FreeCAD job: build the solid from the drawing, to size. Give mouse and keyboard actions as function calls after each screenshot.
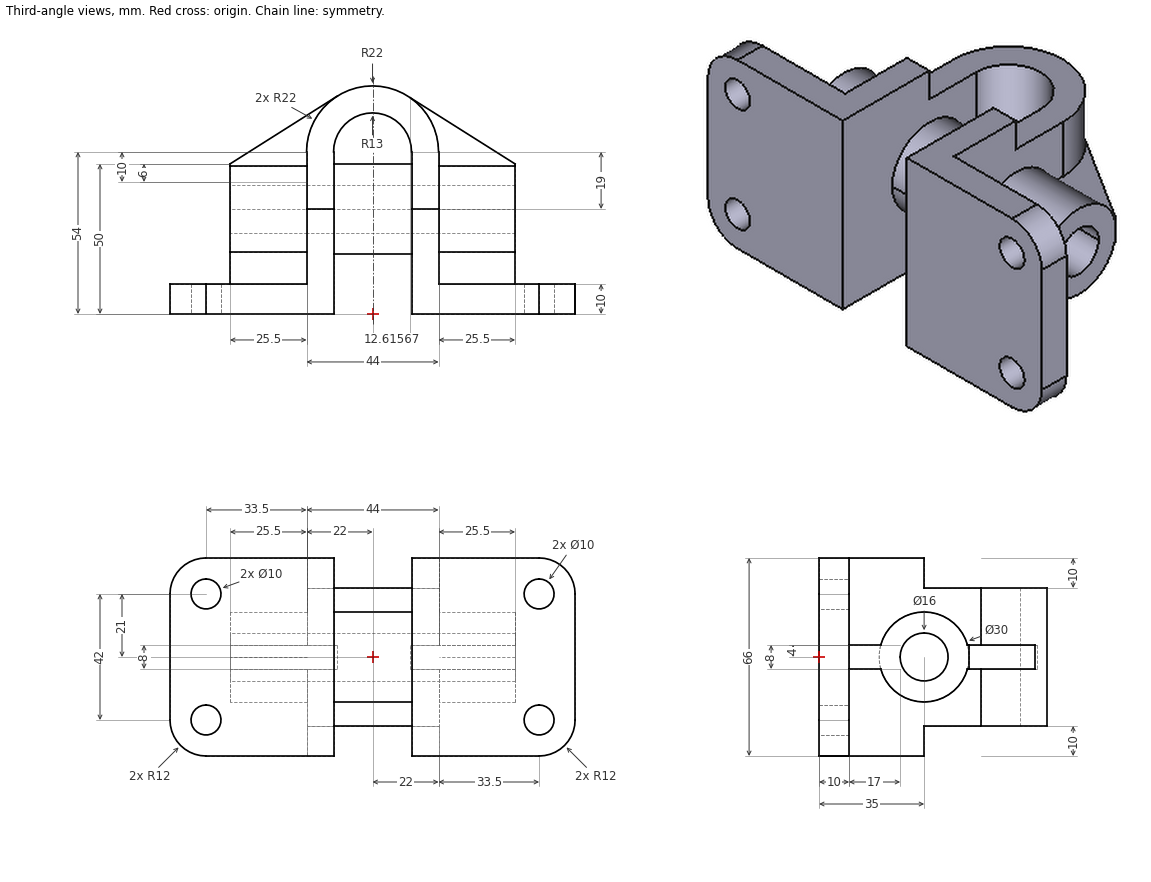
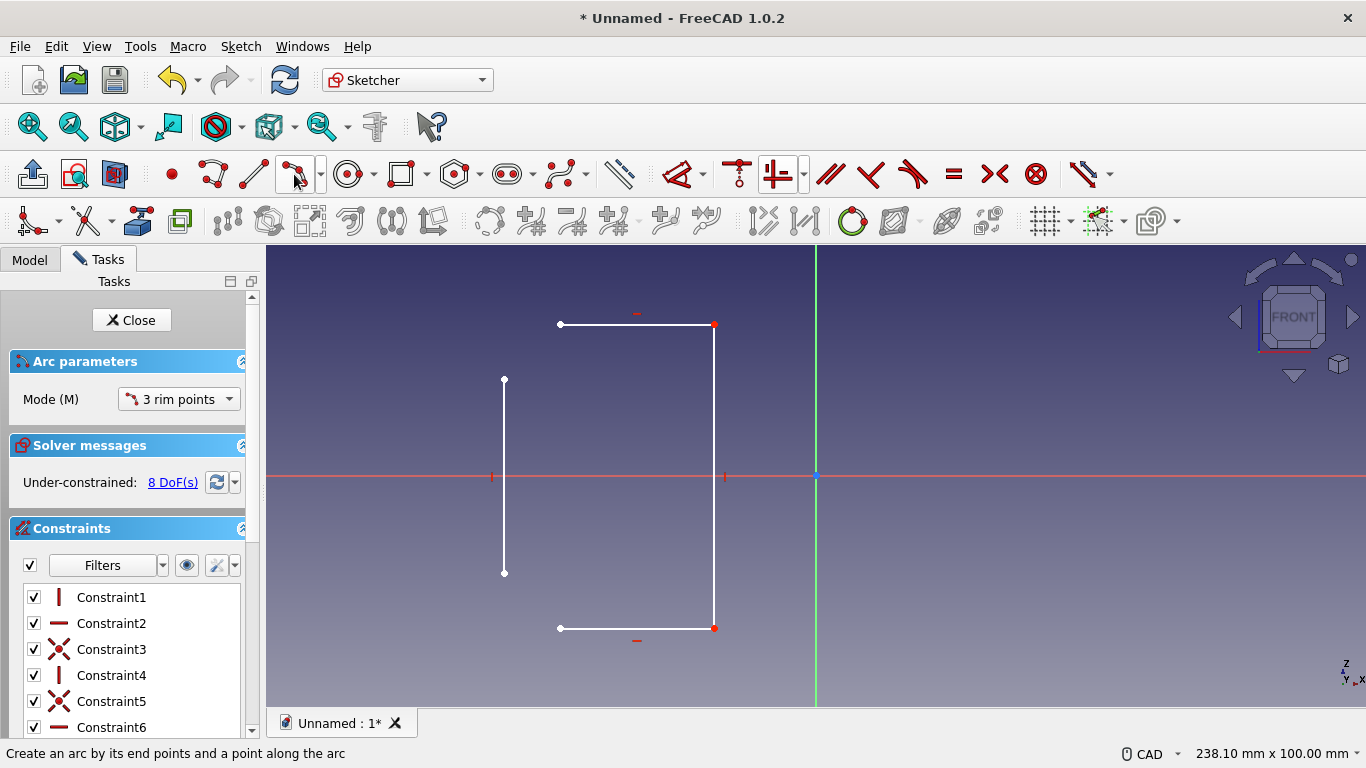
click(504, 380)
click(560, 325)
click(520, 340)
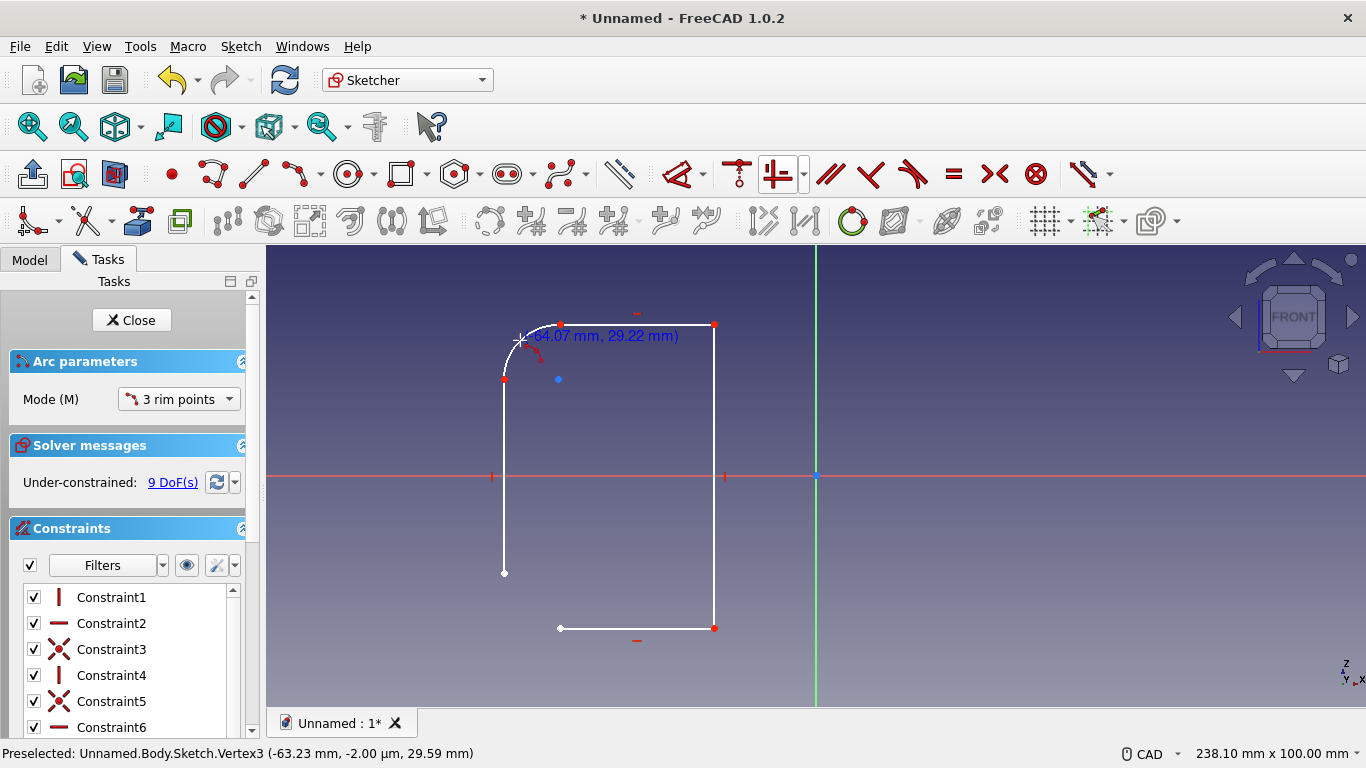
click(560, 629)
click(504, 574)
click(520, 612)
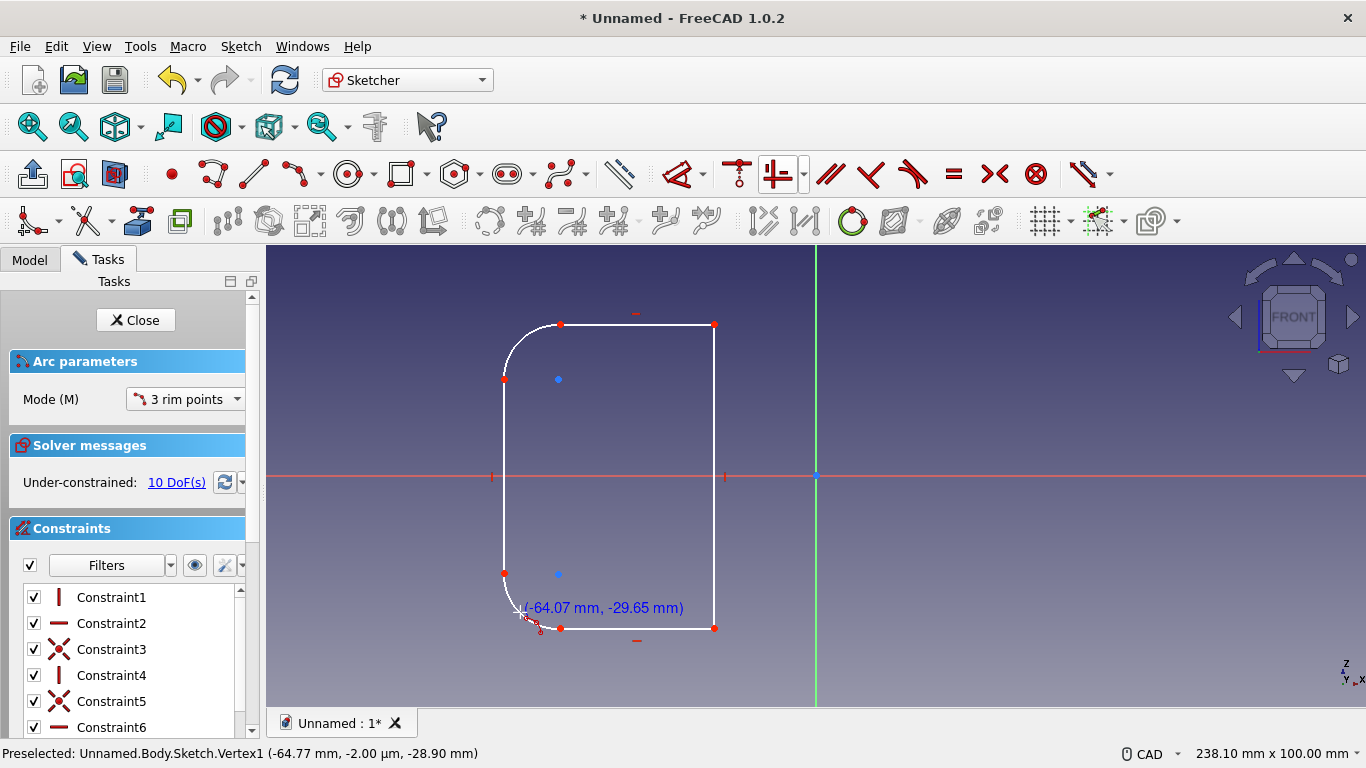
click(348, 174)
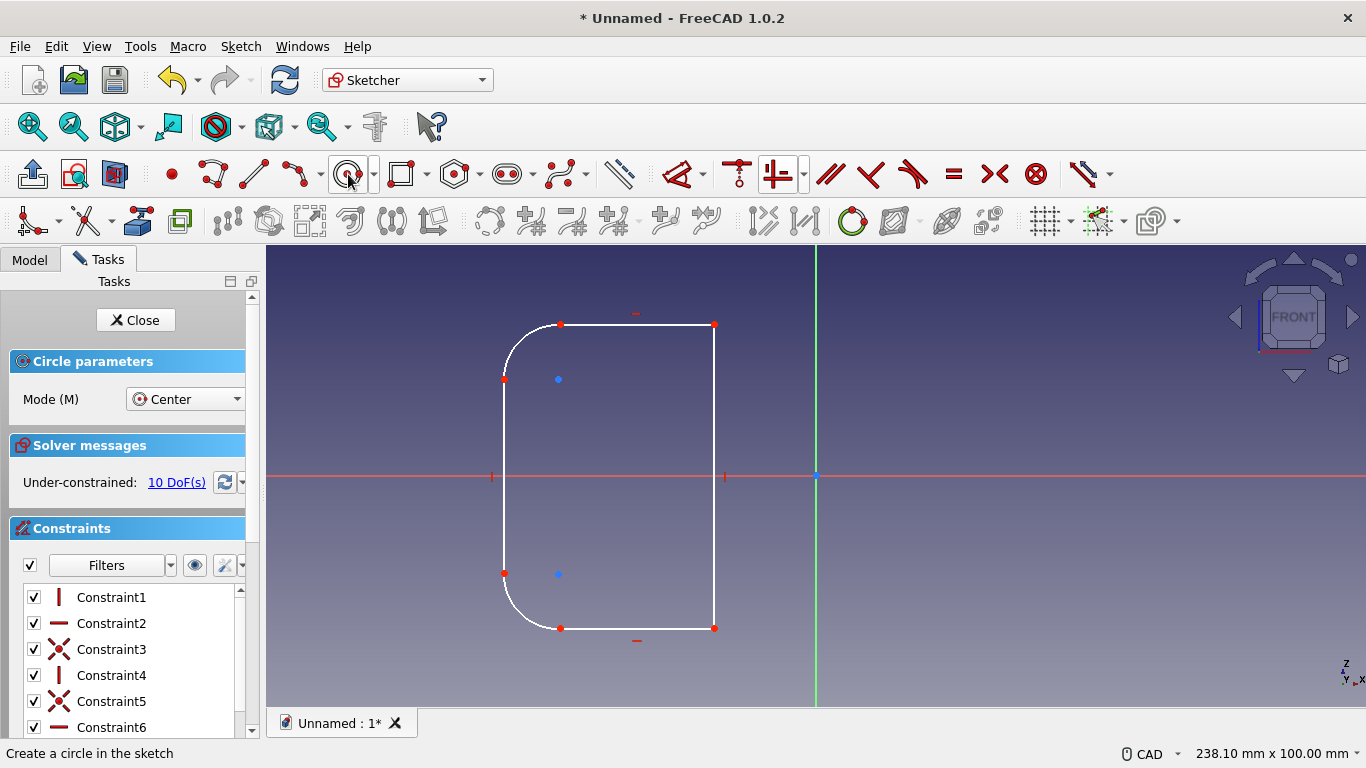
click(560, 379)
move(576, 363)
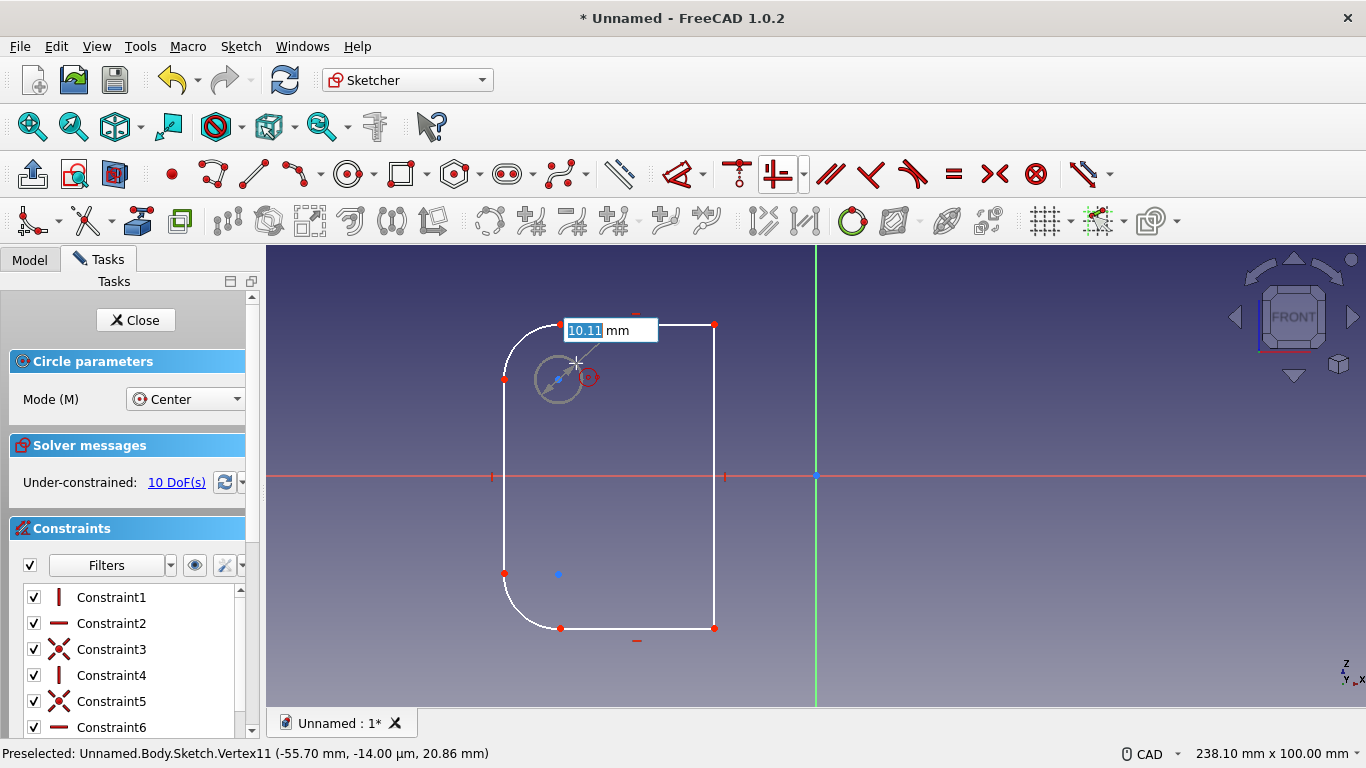
text(10)
key(Return)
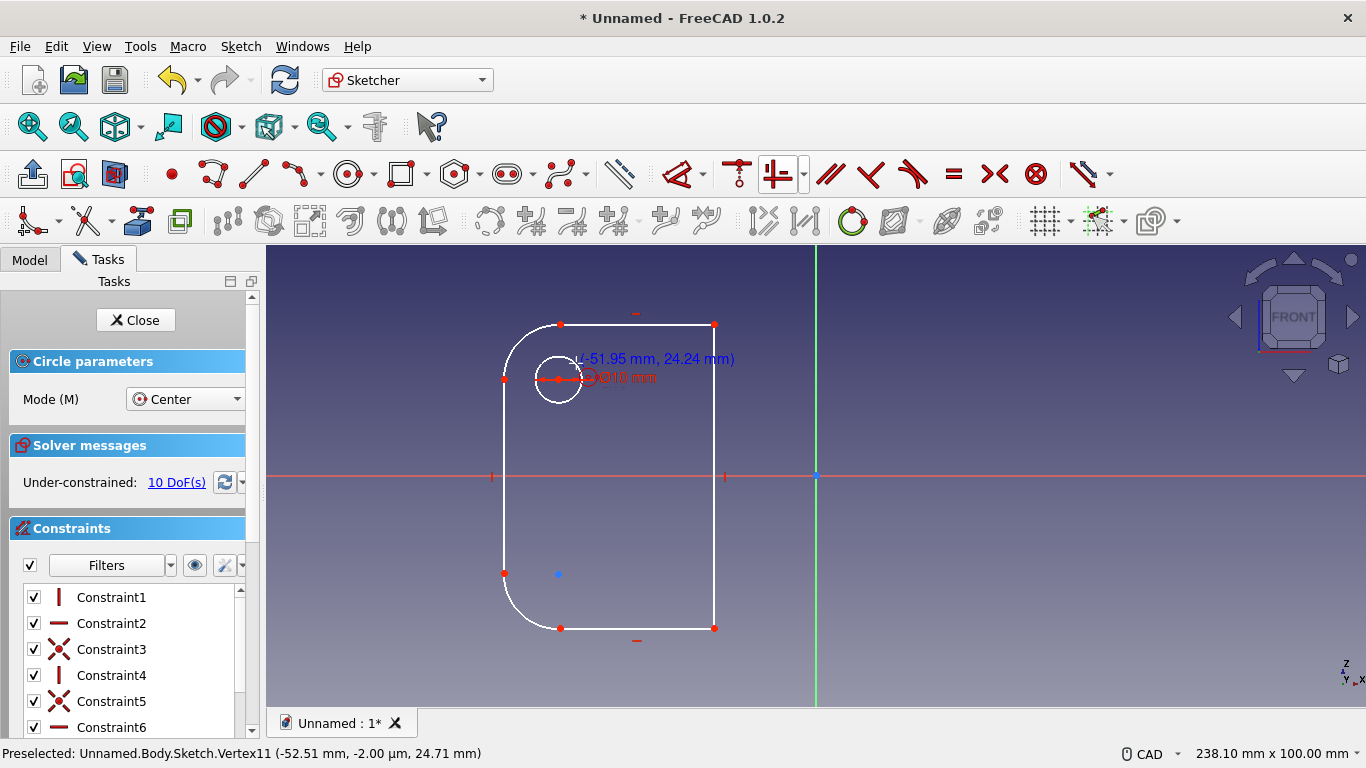
click(560, 573)
move(576, 557)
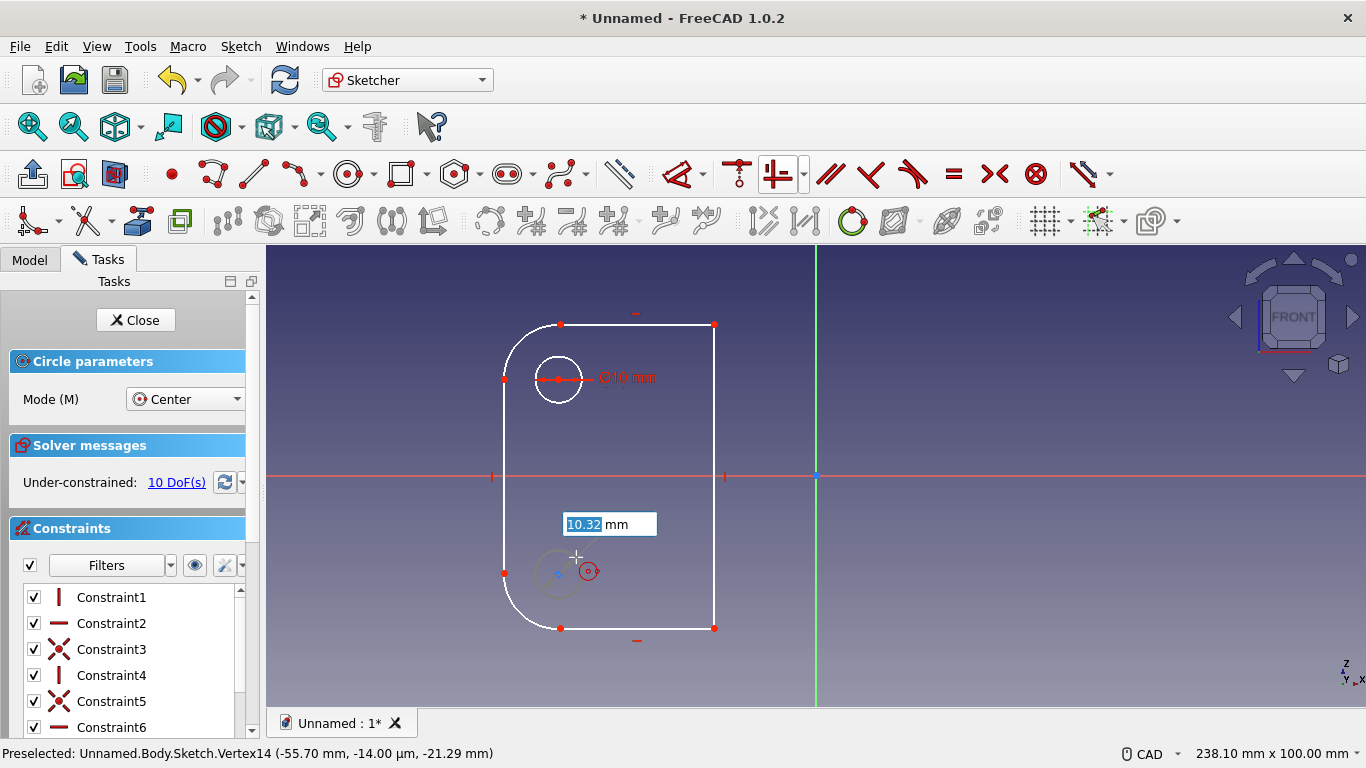
text(10)
key(Return)
key(Escape)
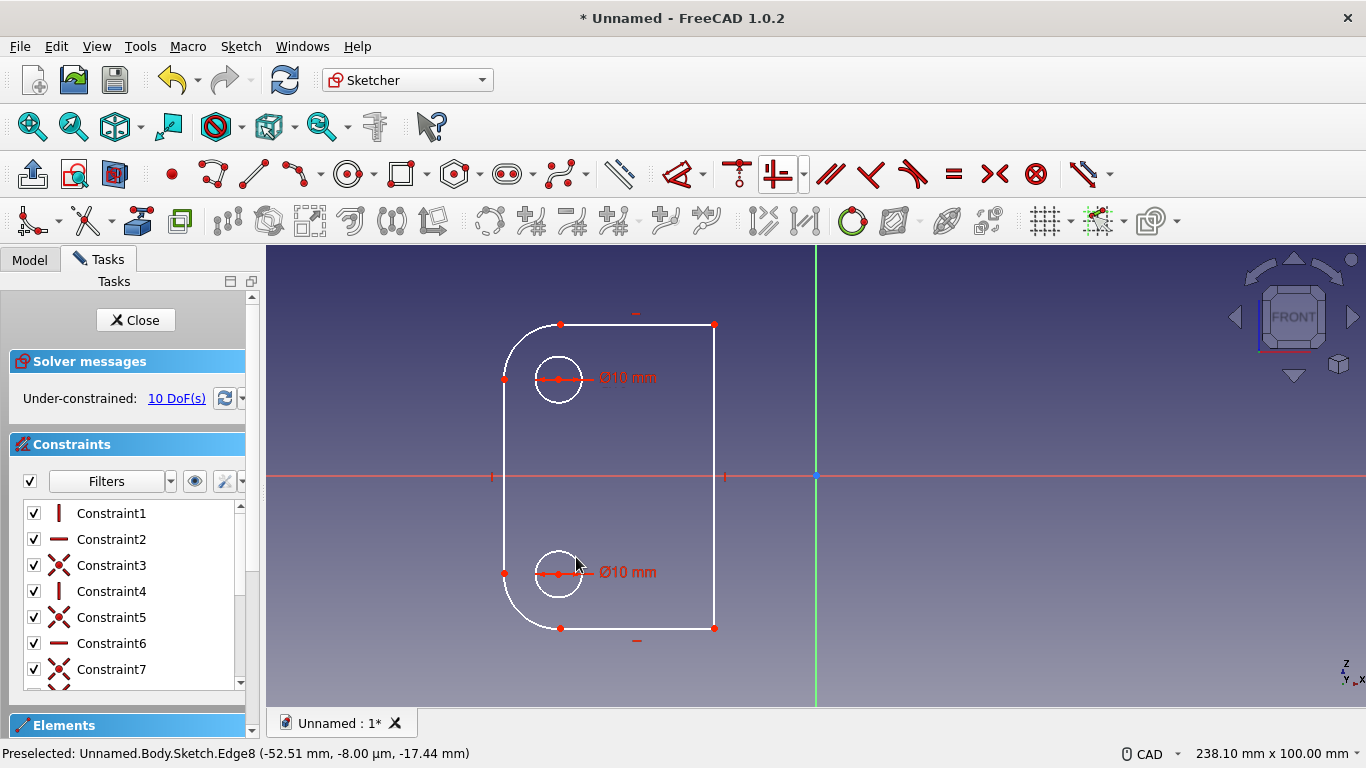
click(504, 516)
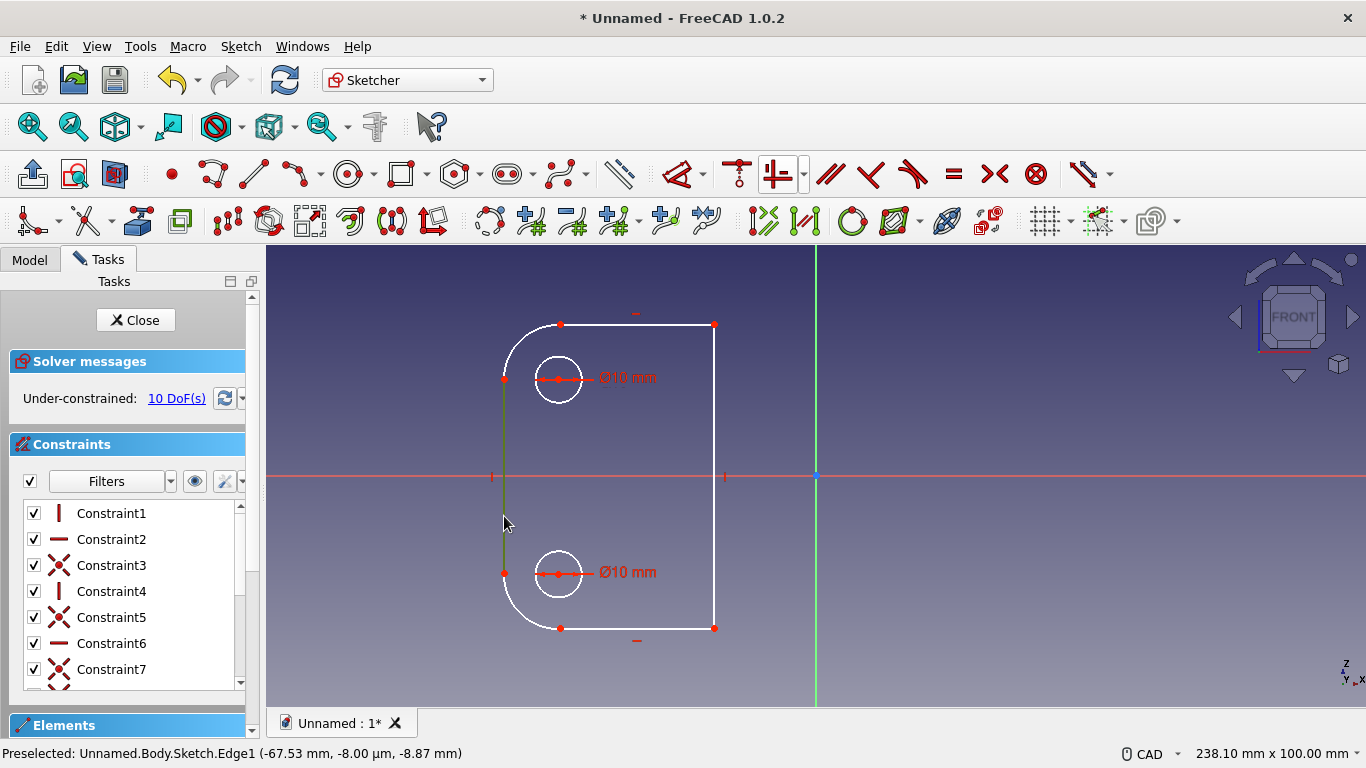
click(535, 331)